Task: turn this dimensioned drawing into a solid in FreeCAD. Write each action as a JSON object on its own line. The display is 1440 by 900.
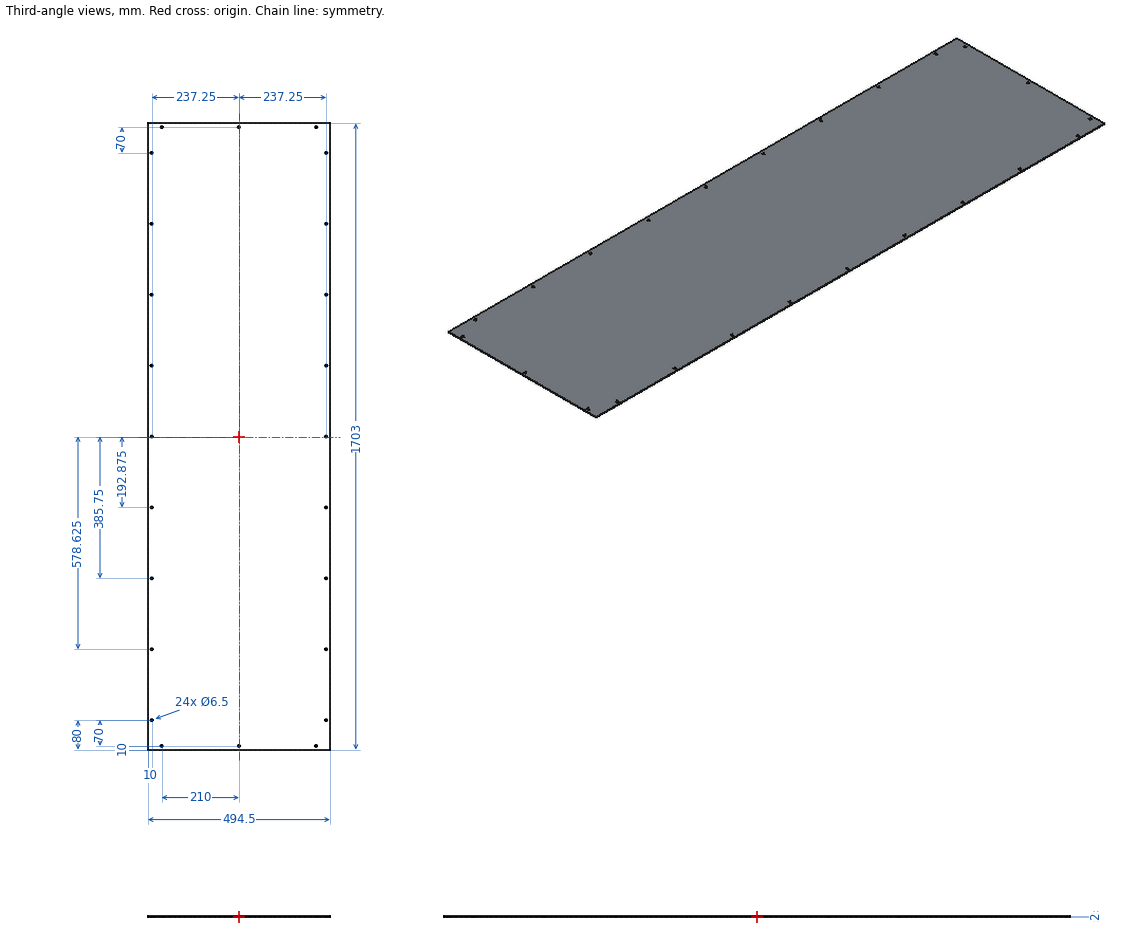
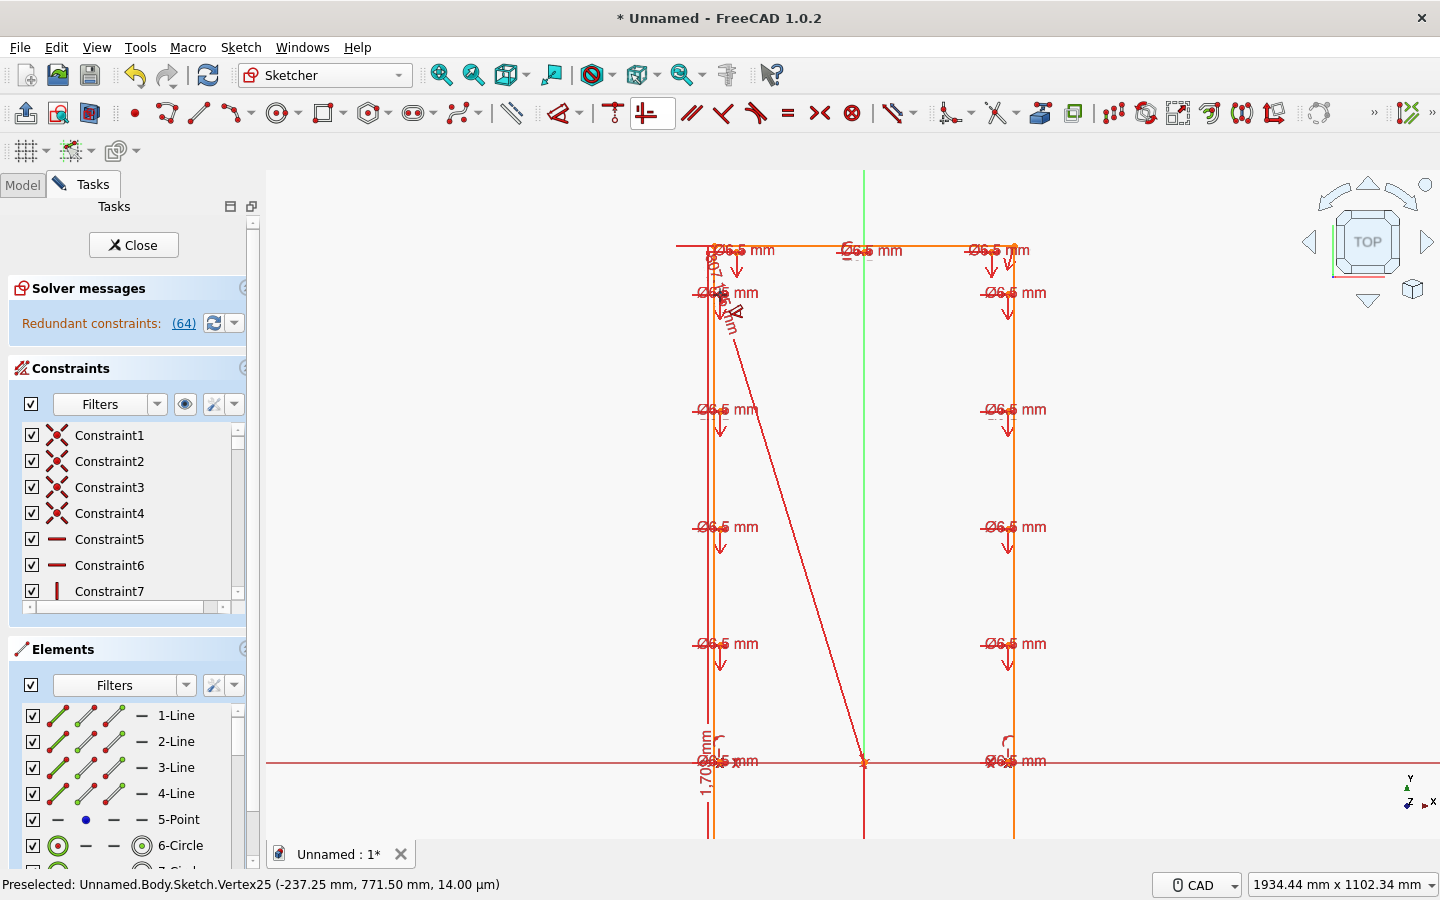
{"action": "left_click", "coordinate": [864, 253]}
{"action": "left_click", "coordinate": [686, 274]}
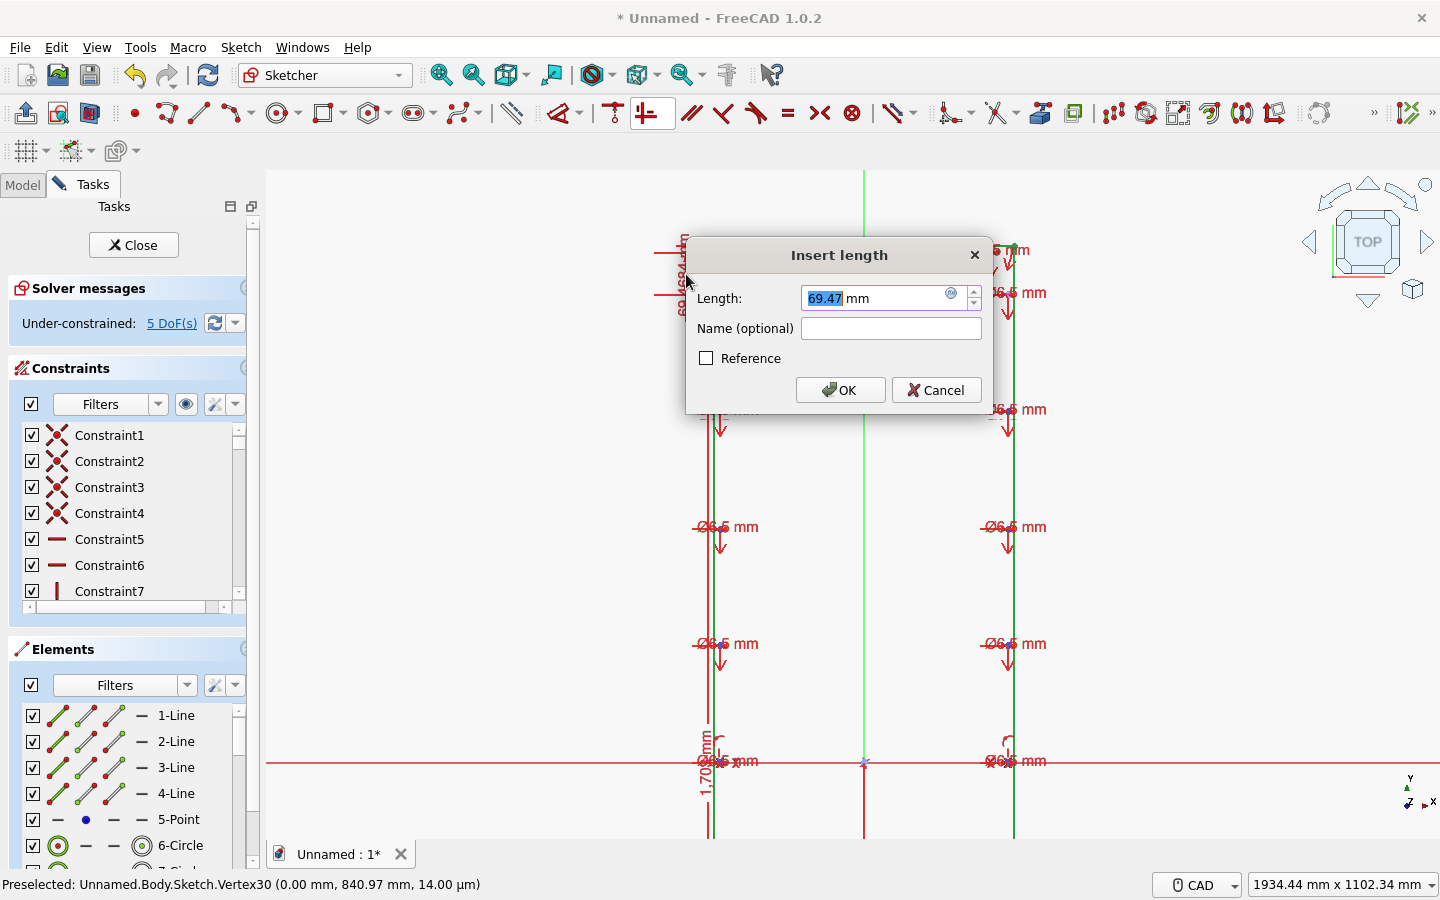
{"action": "type", "text": "70"}
{"action": "key", "text": "Return"}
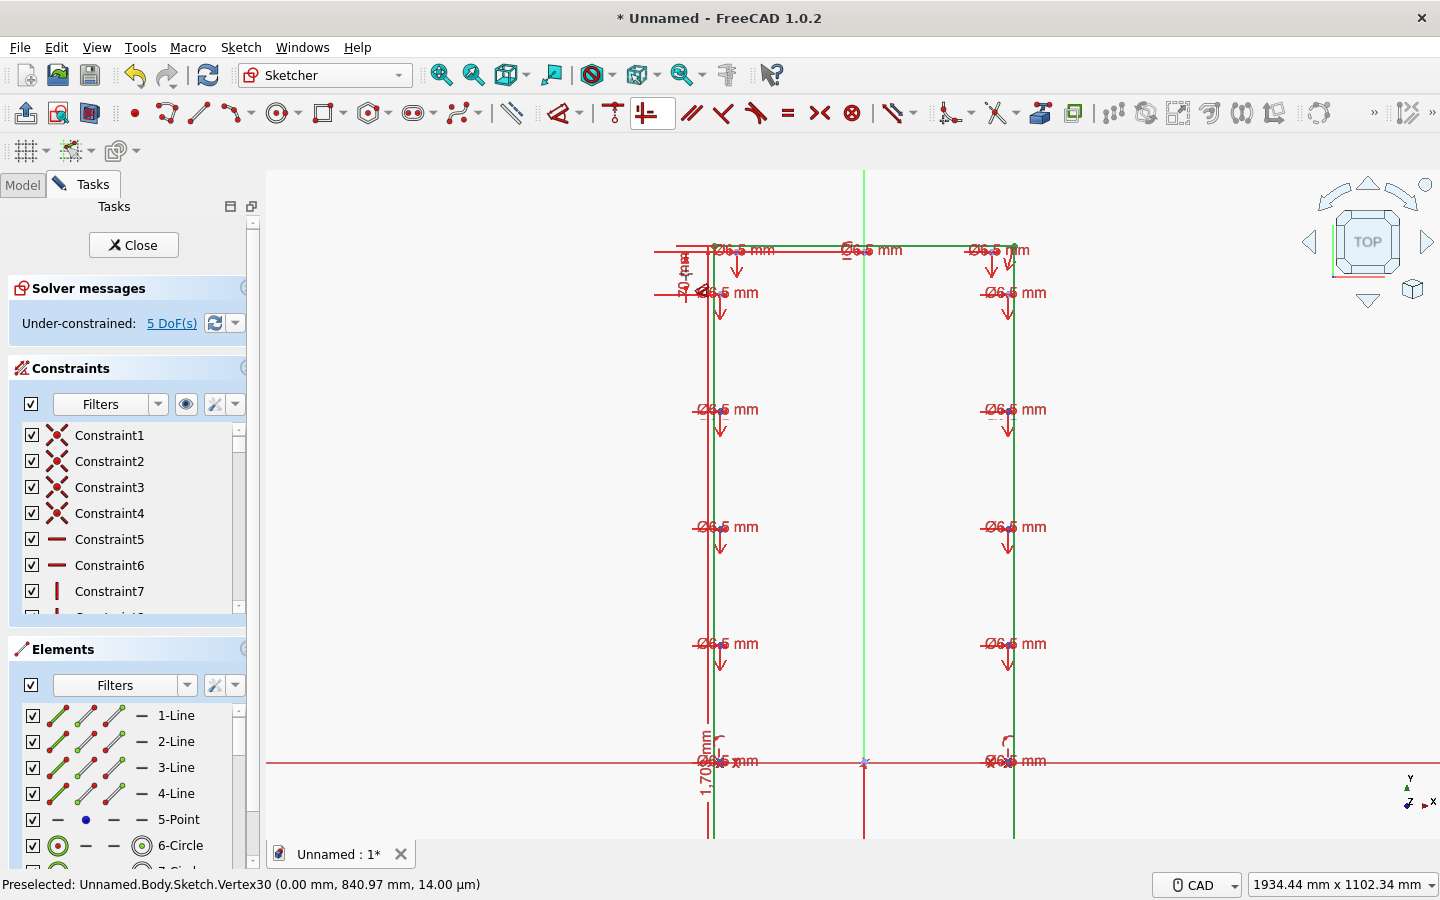
{"action": "scroll", "coordinate": [720, 294], "scroll_direction": "down", "scroll_amount": 4}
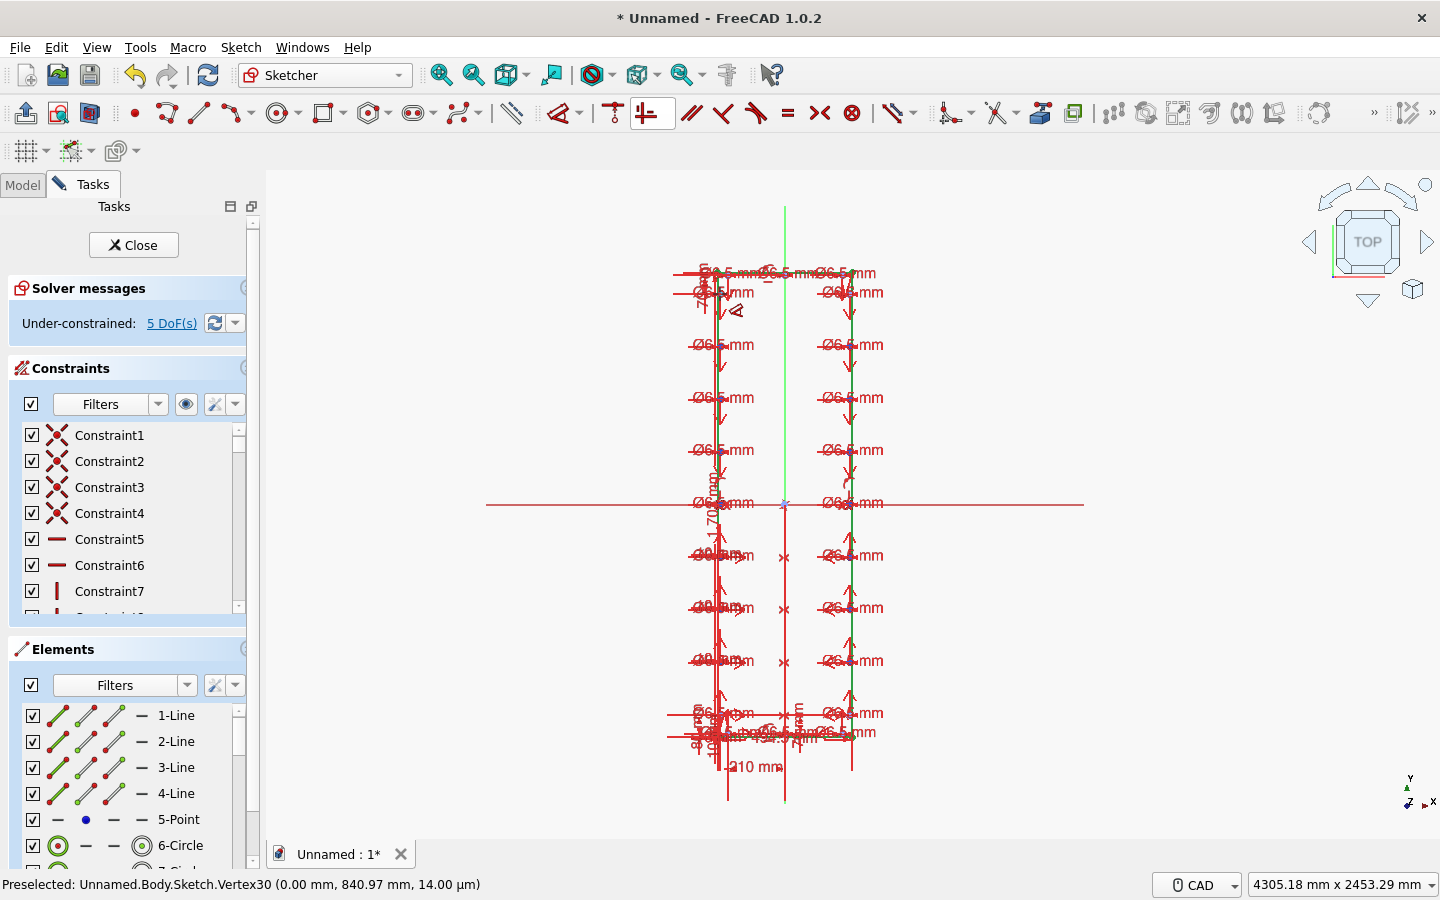
{"action": "left_click", "coordinate": [720, 610]}
{"action": "left_click", "coordinate": [686, 533]}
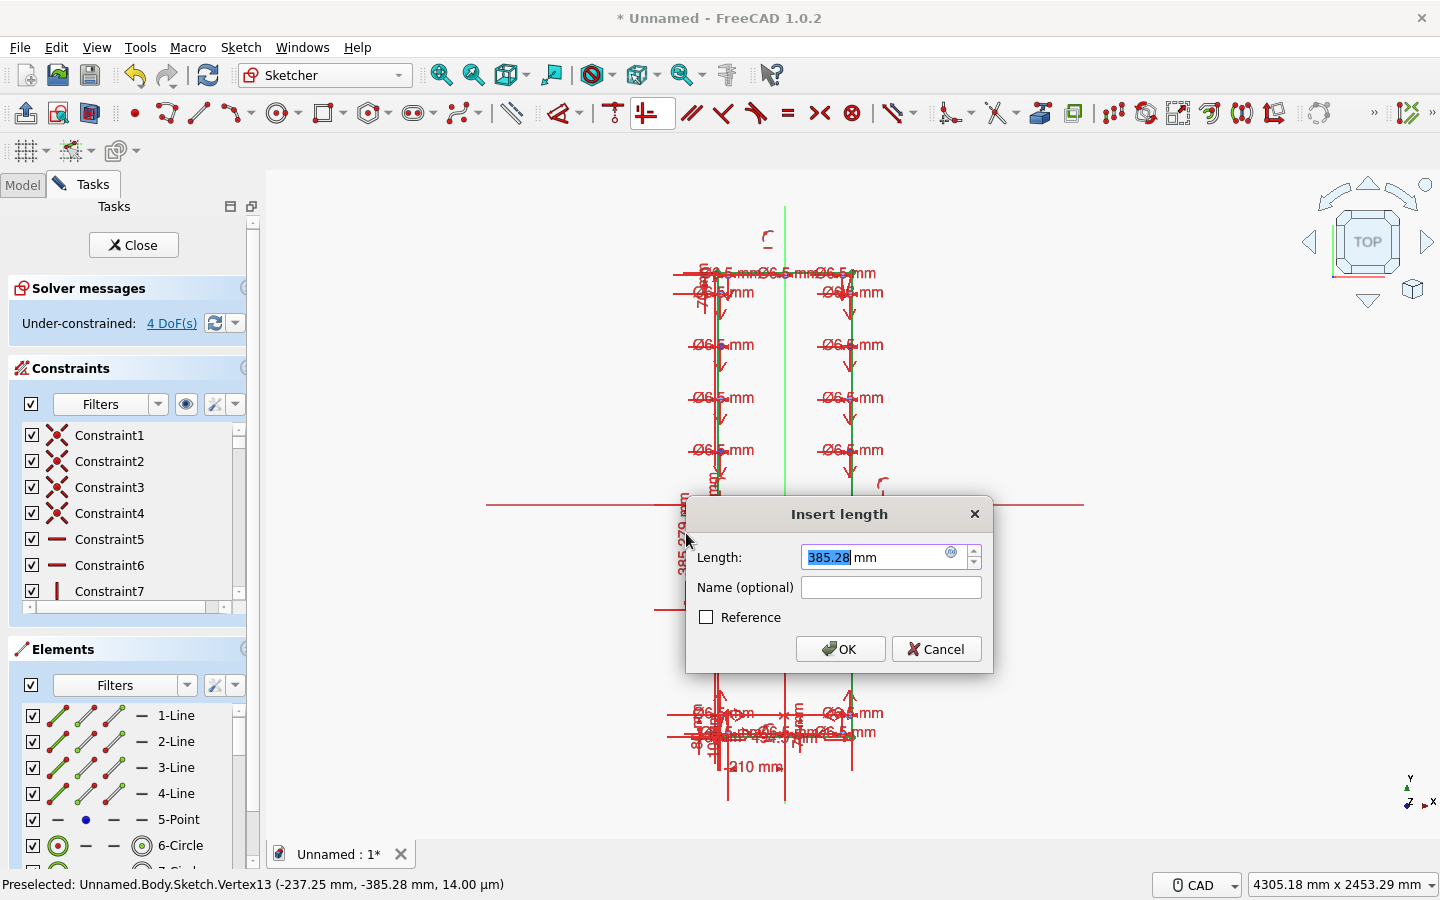
{"action": "type", "text": "385.75"}
{"action": "key", "text": "Return"}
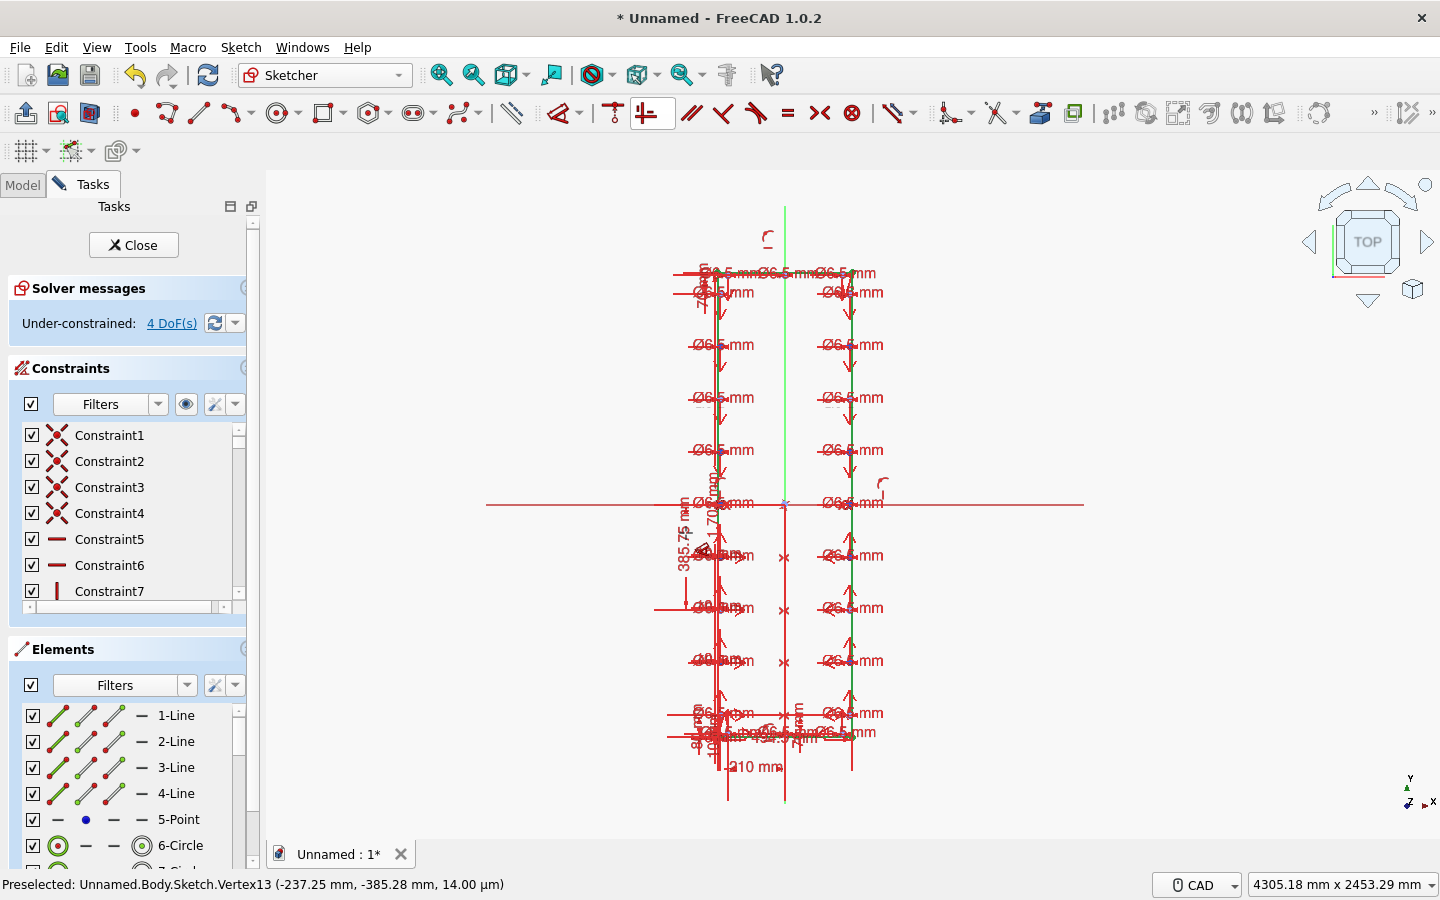
{"action": "left_click", "coordinate": [720, 505]}
{"action": "left_click", "coordinate": [753, 471]}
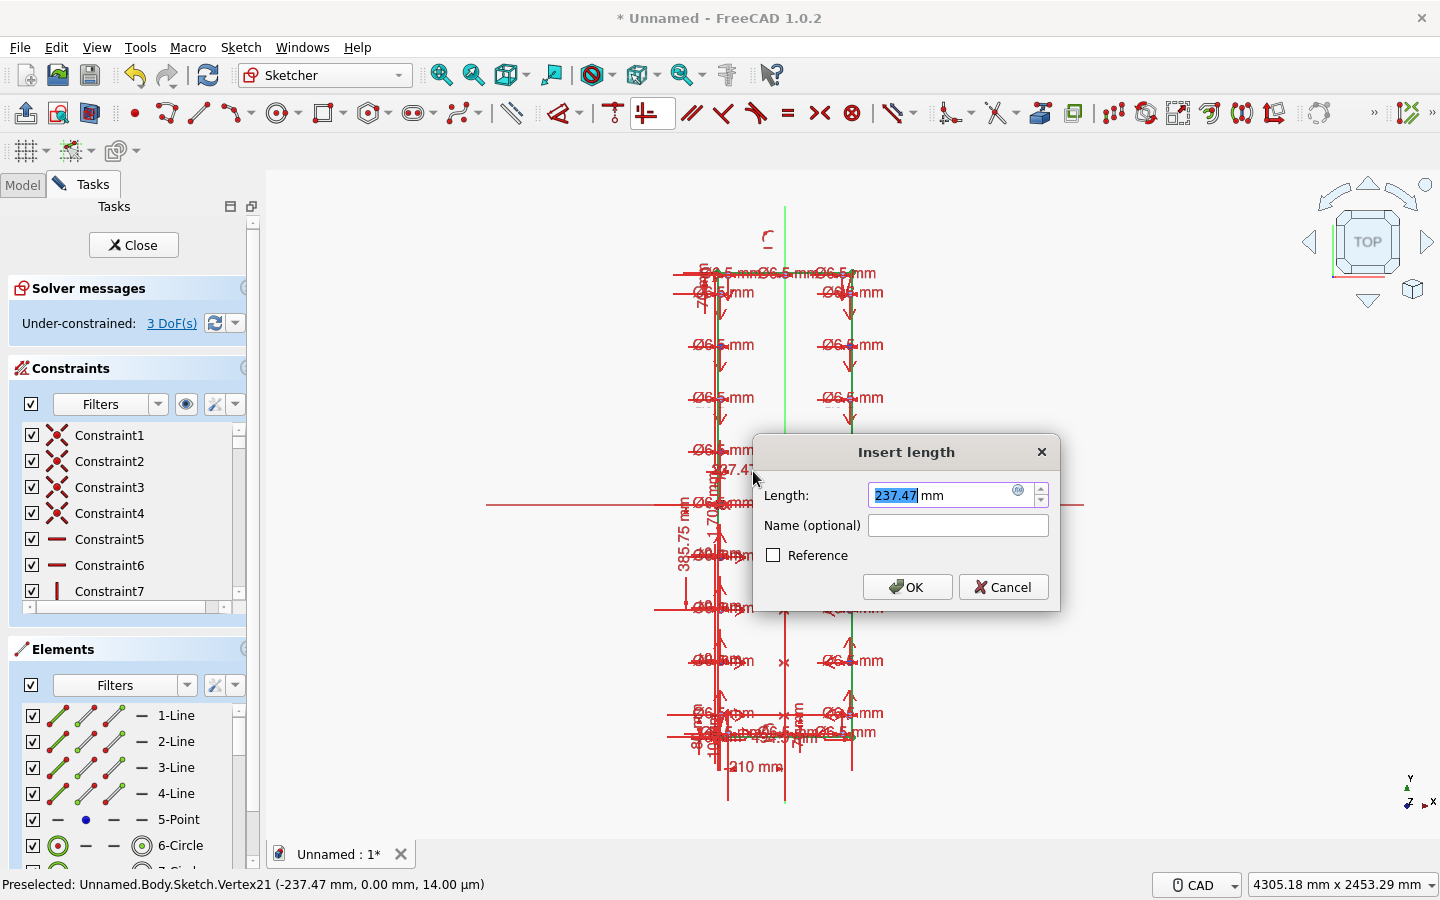
{"action": "type", "text": "237.25"}
{"action": "key", "text": "Return"}